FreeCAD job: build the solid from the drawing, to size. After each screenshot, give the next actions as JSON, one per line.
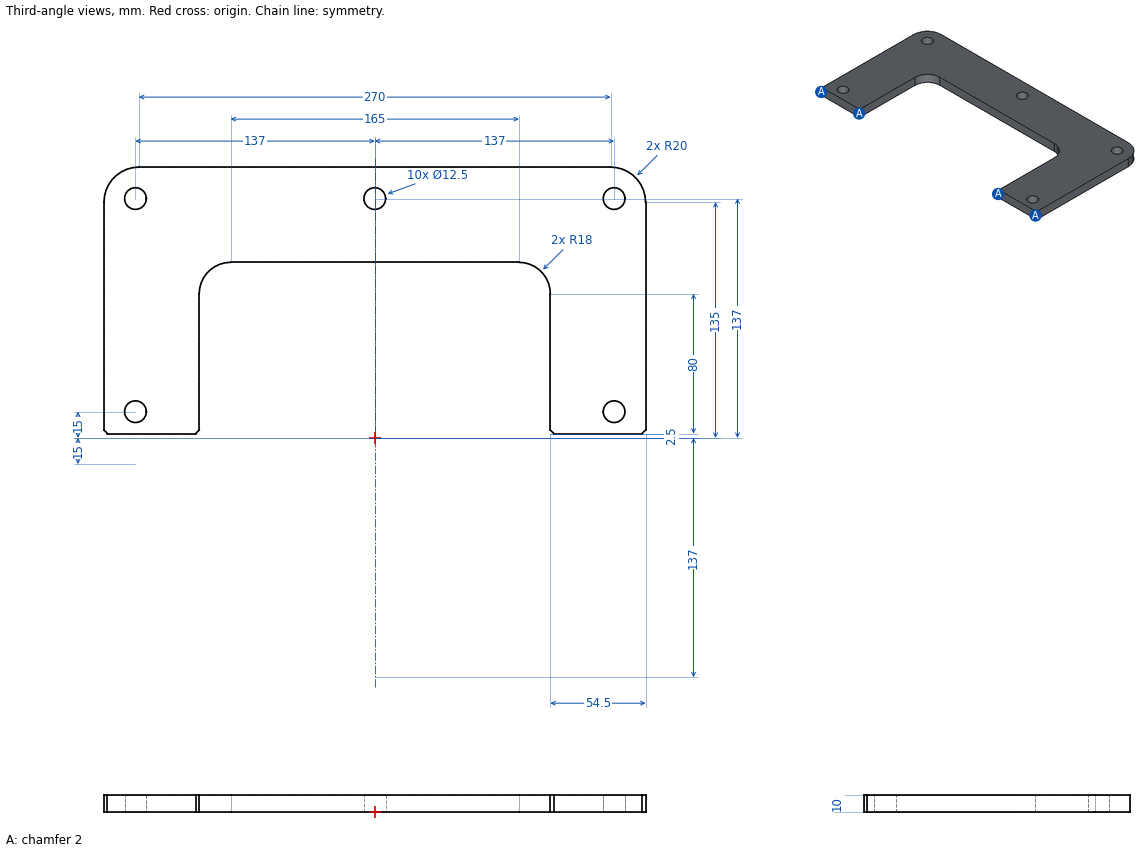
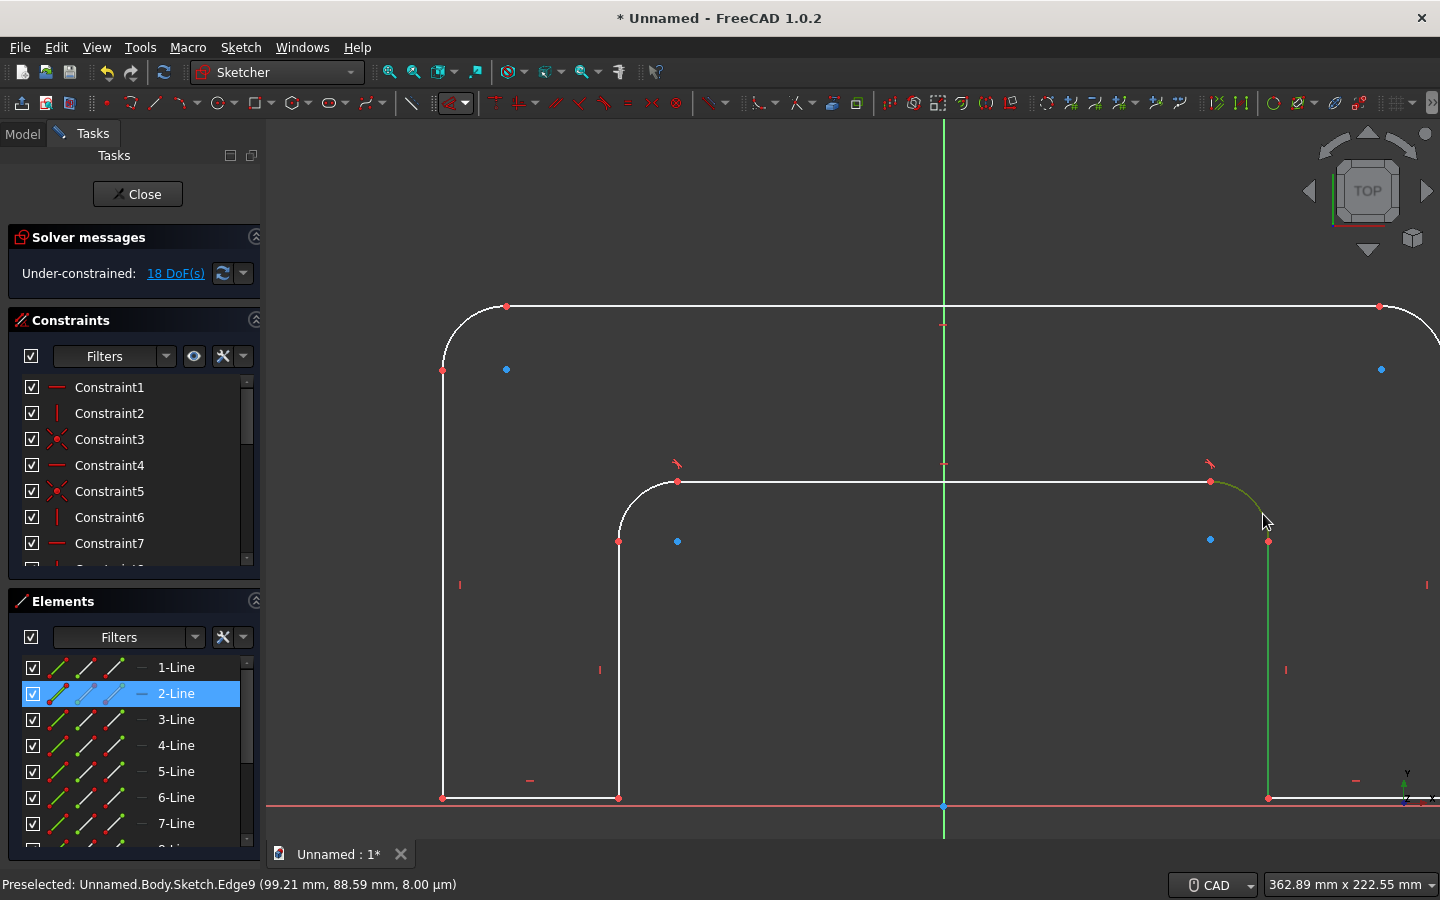
{"action": "key", "text": "t"}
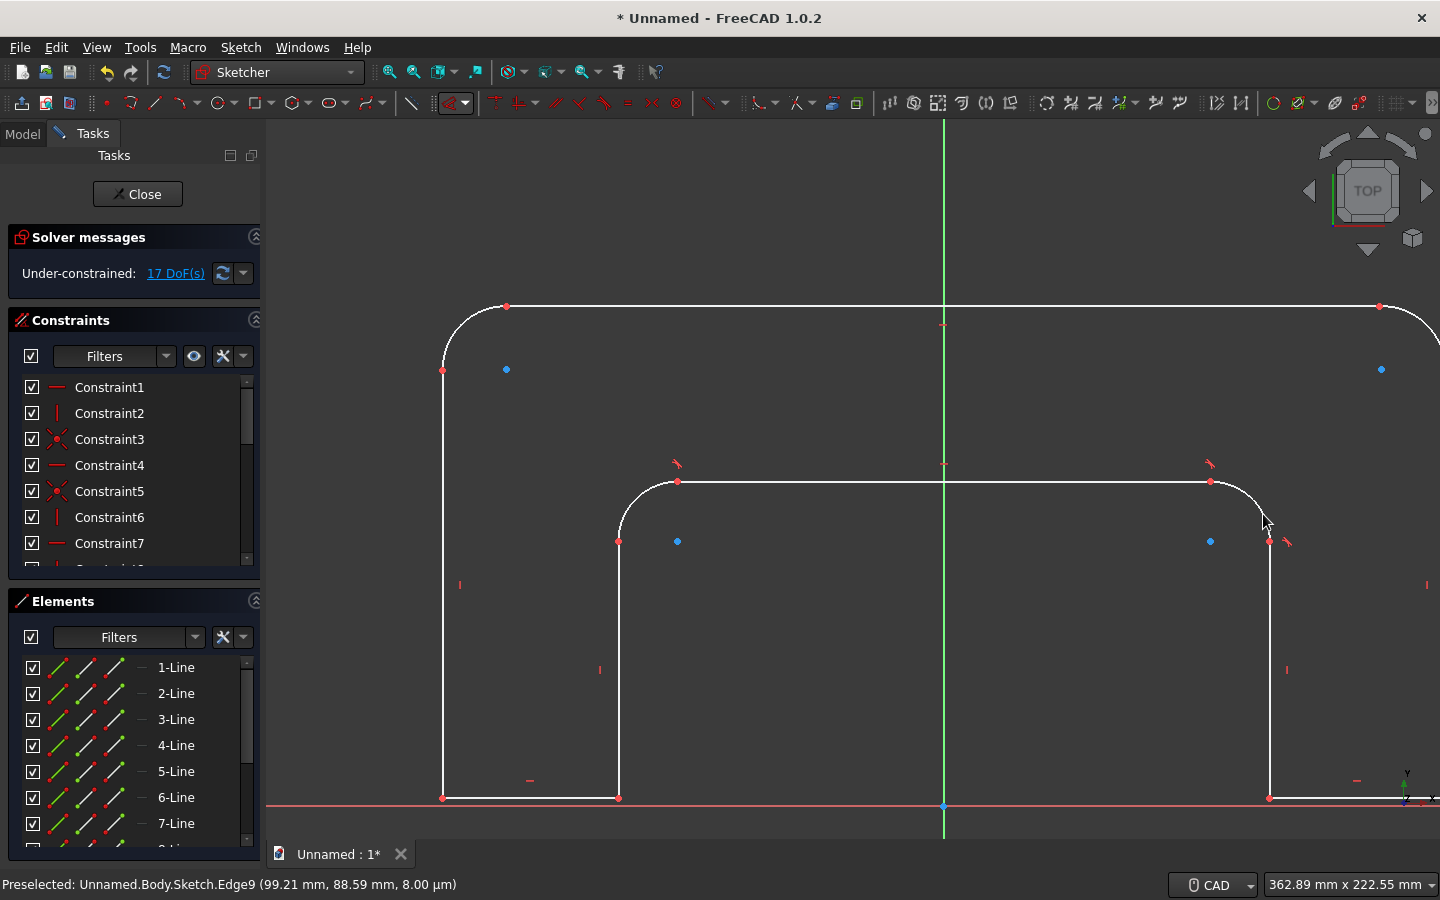
{"action": "scroll", "coordinate": [461, 324], "scroll_direction": "down", "scroll_amount": 2}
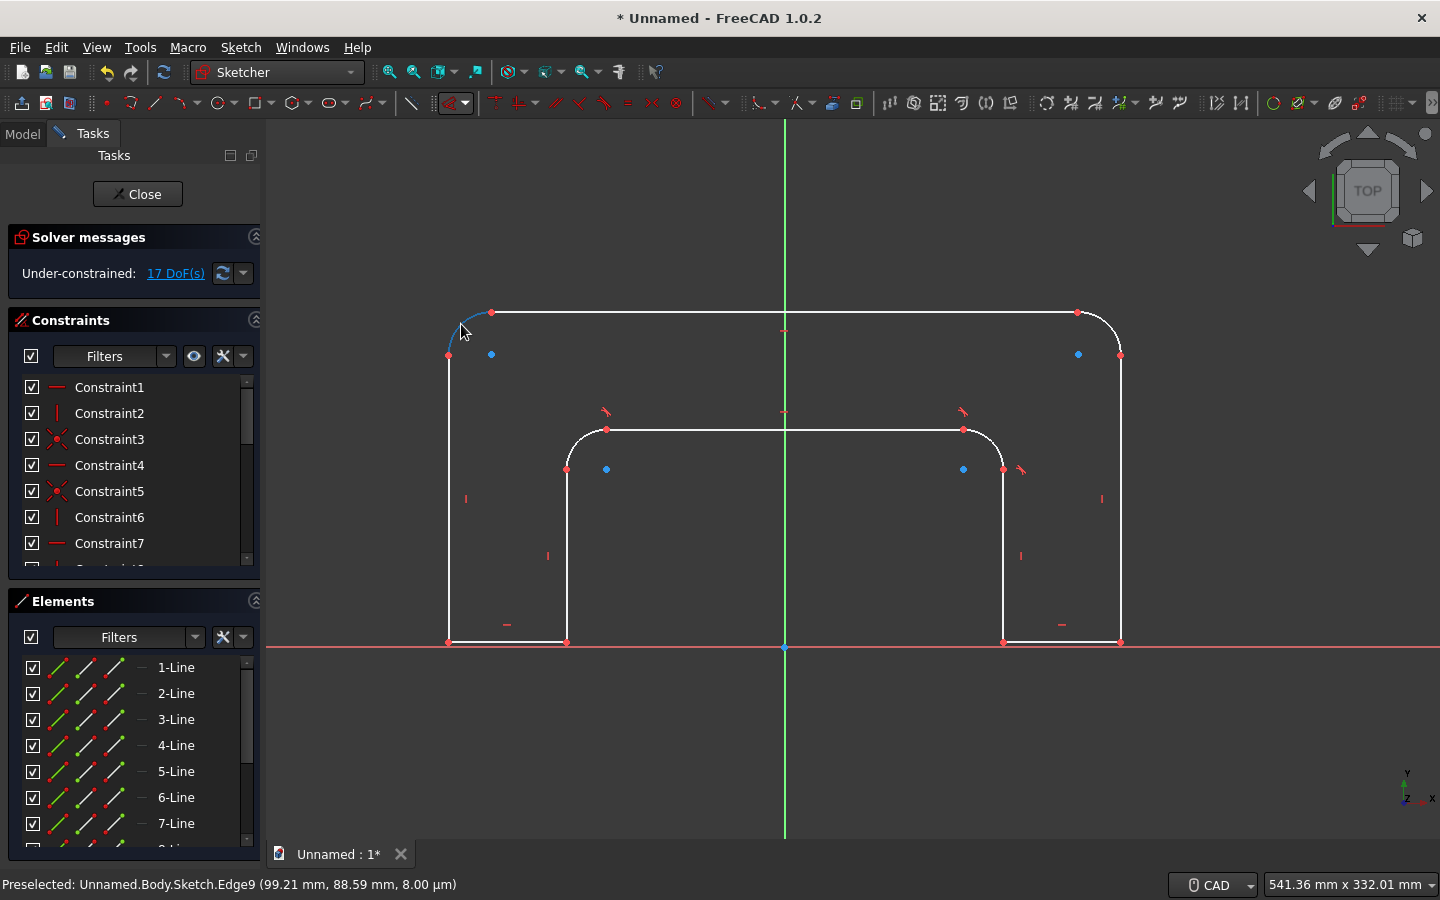
{"action": "left_click", "coordinate": [1121, 556]}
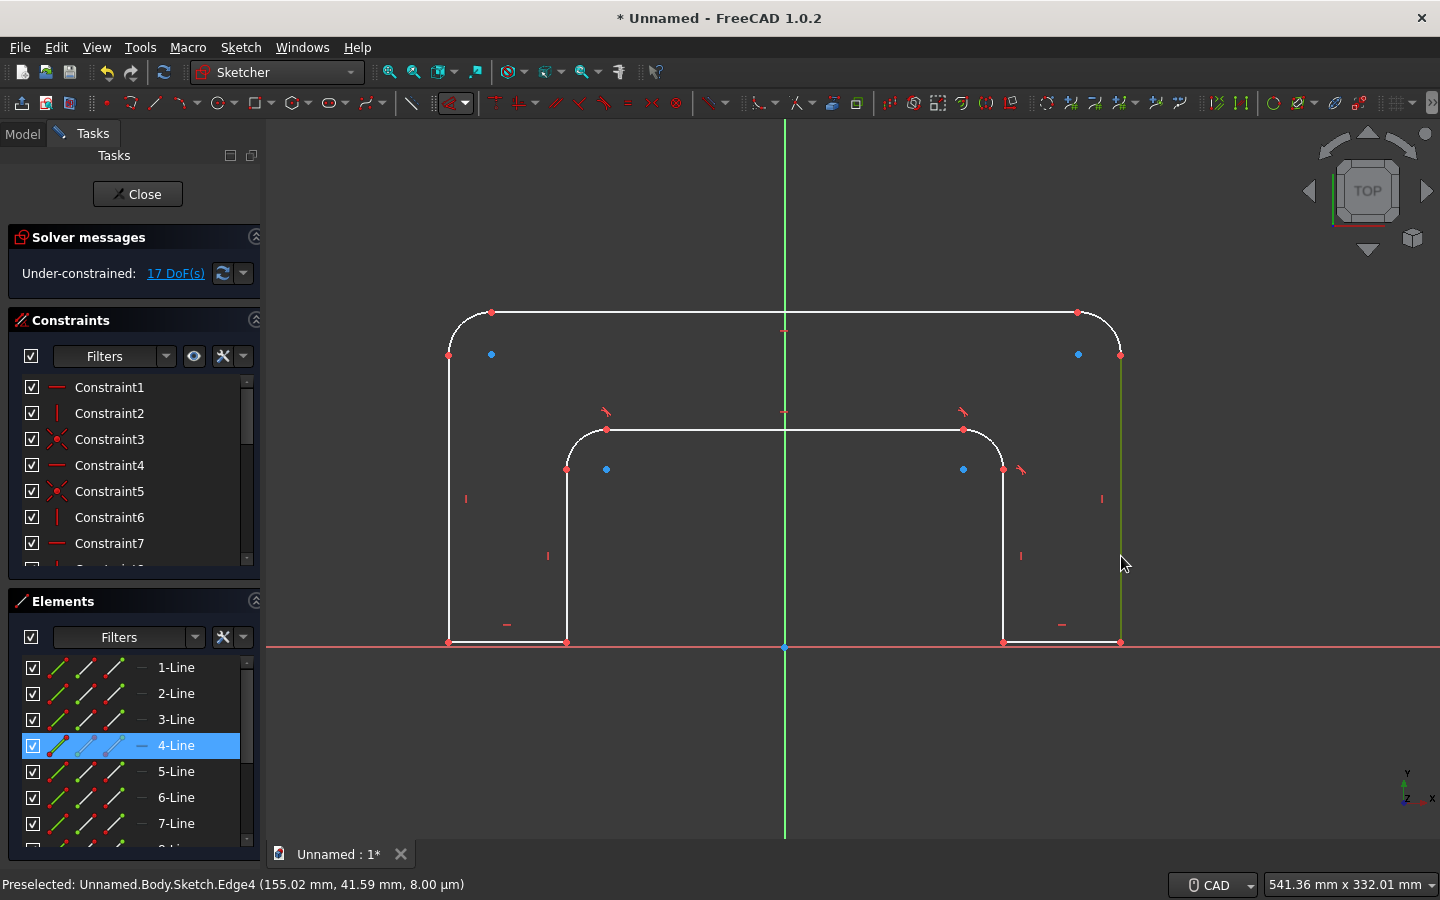
{"action": "left_click", "coordinate": [1116, 335]}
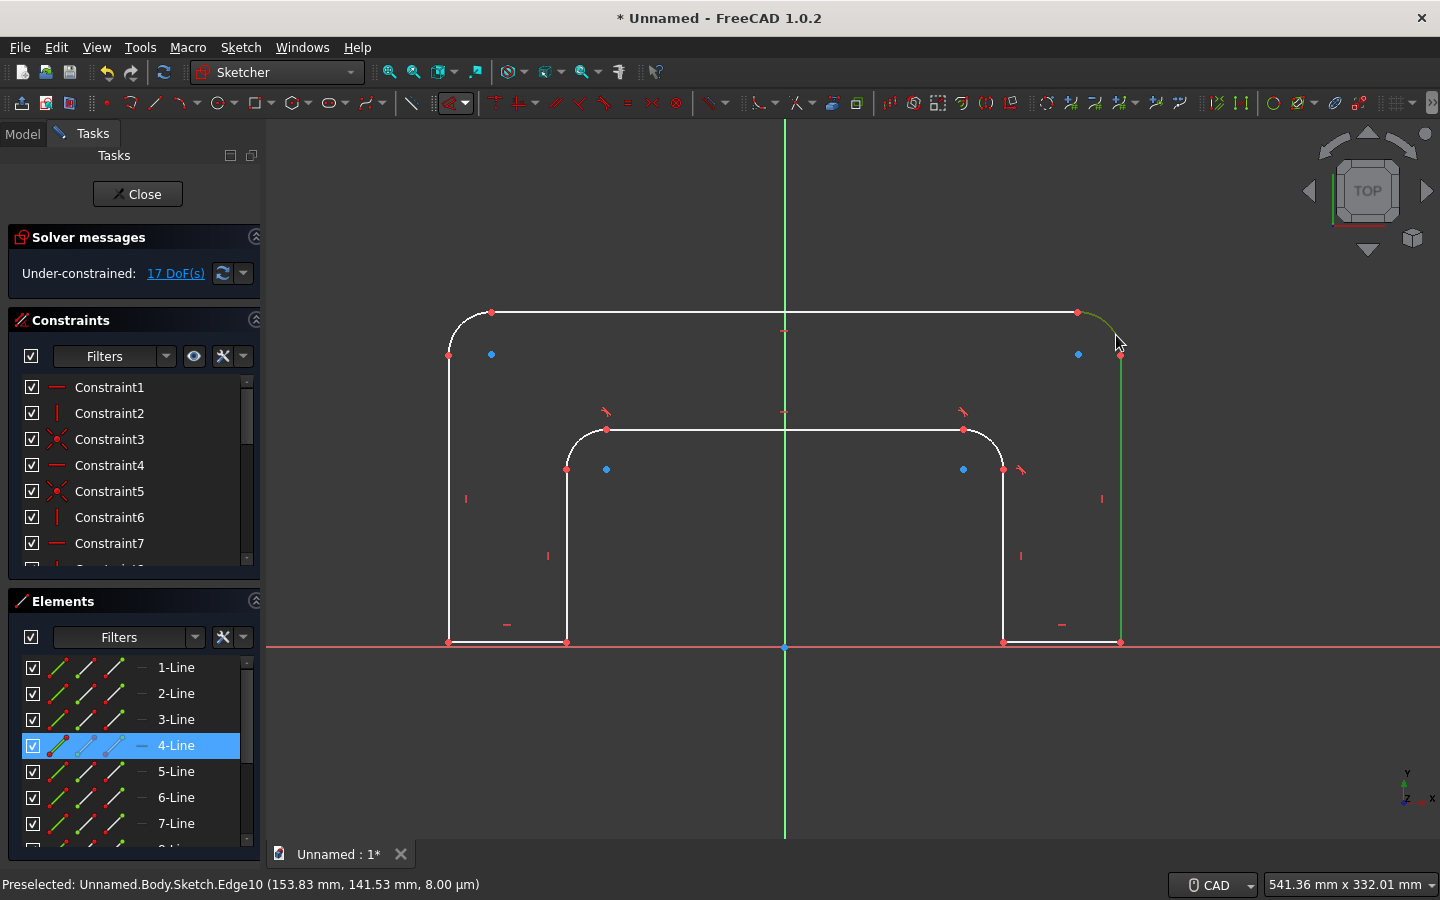
{"action": "key", "text": "t"}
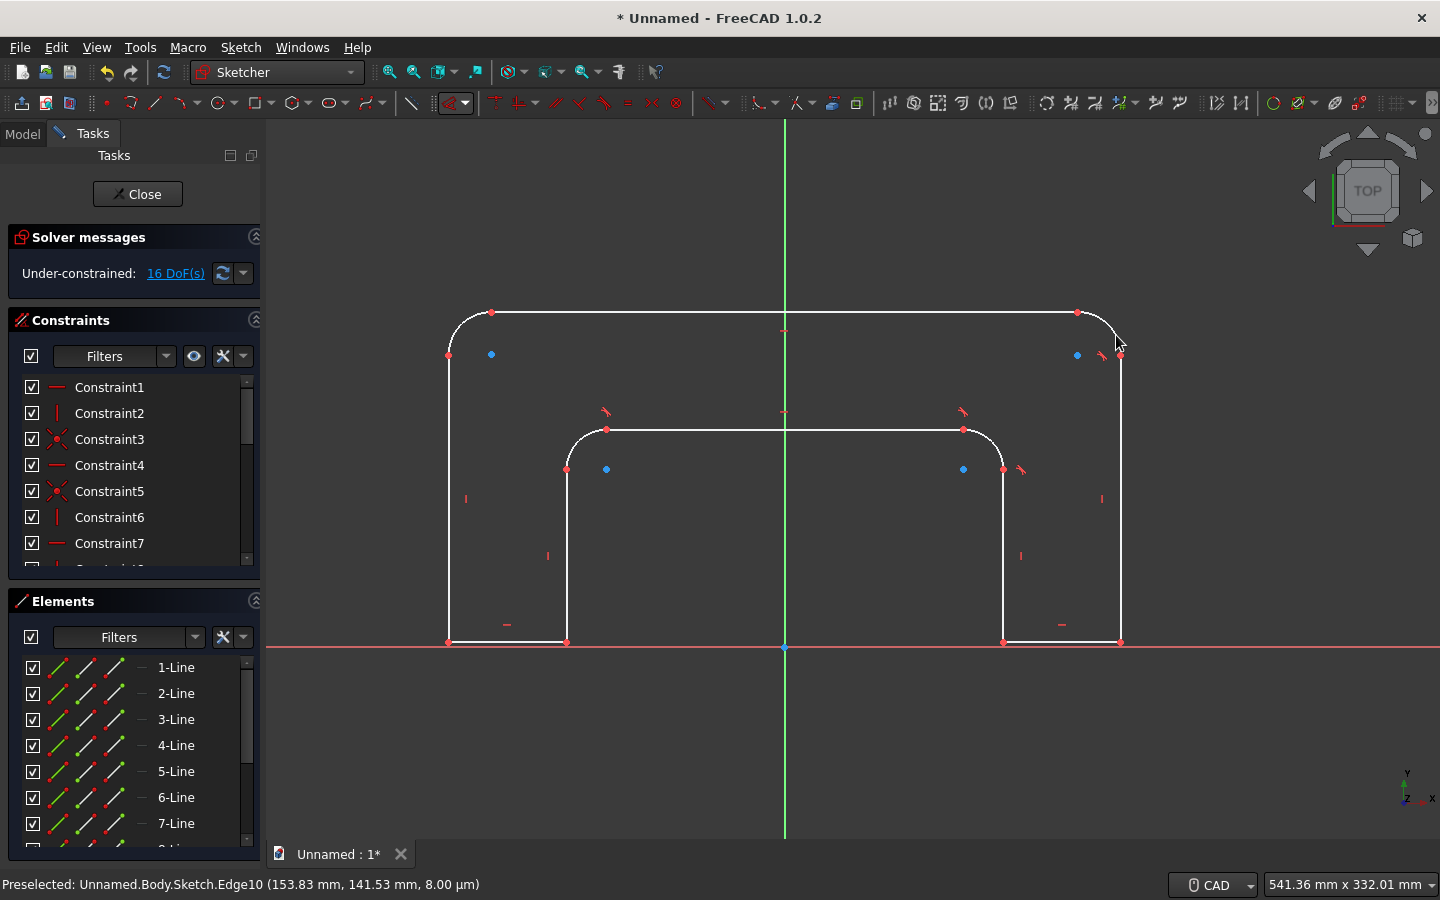
{"action": "left_click", "coordinate": [901, 312]}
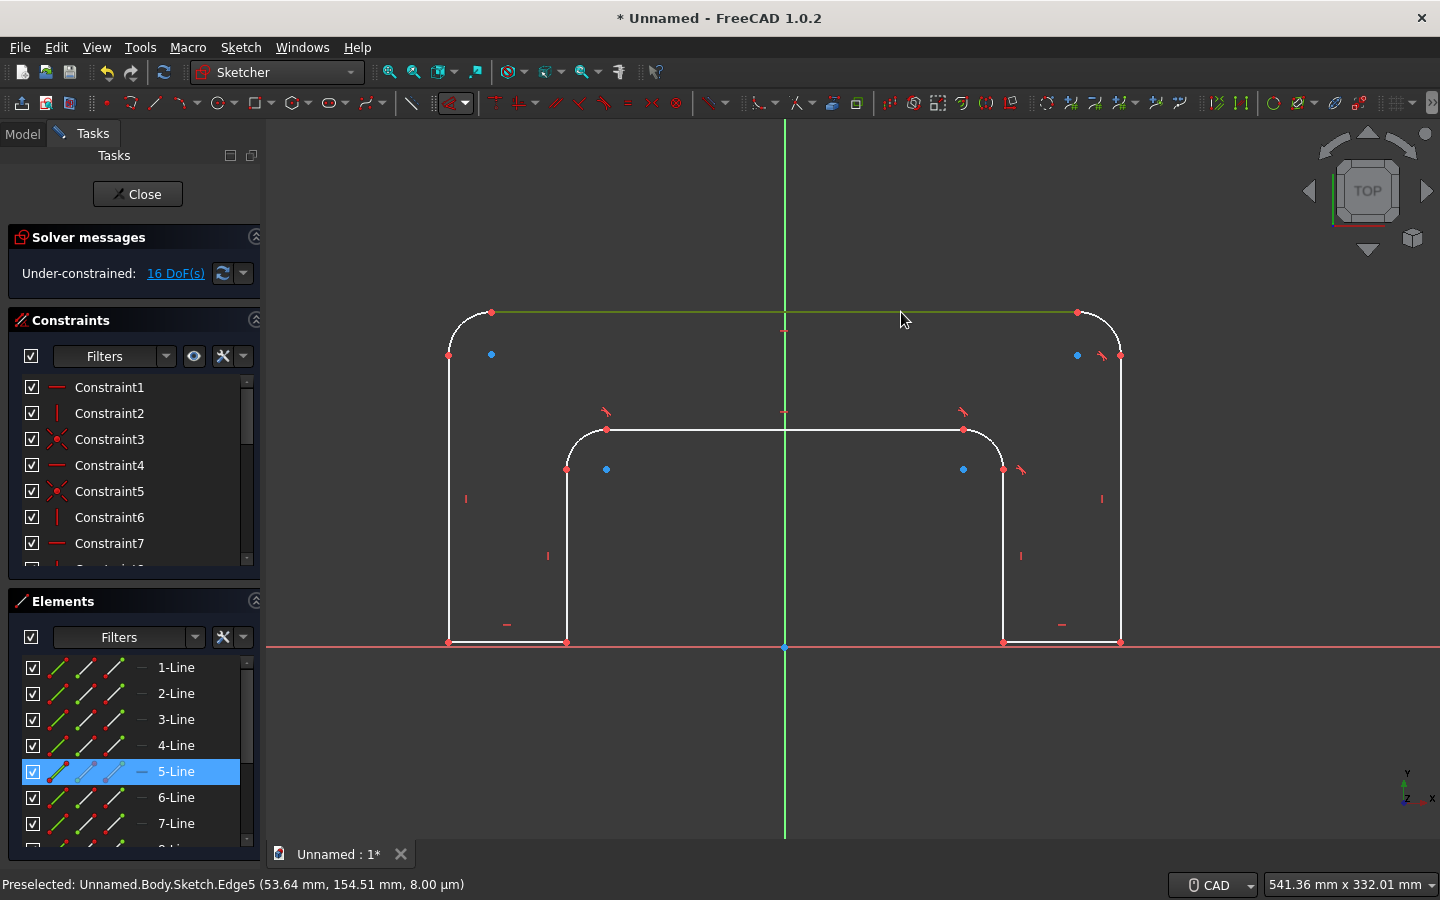
{"action": "left_click", "coordinate": [1116, 335]}